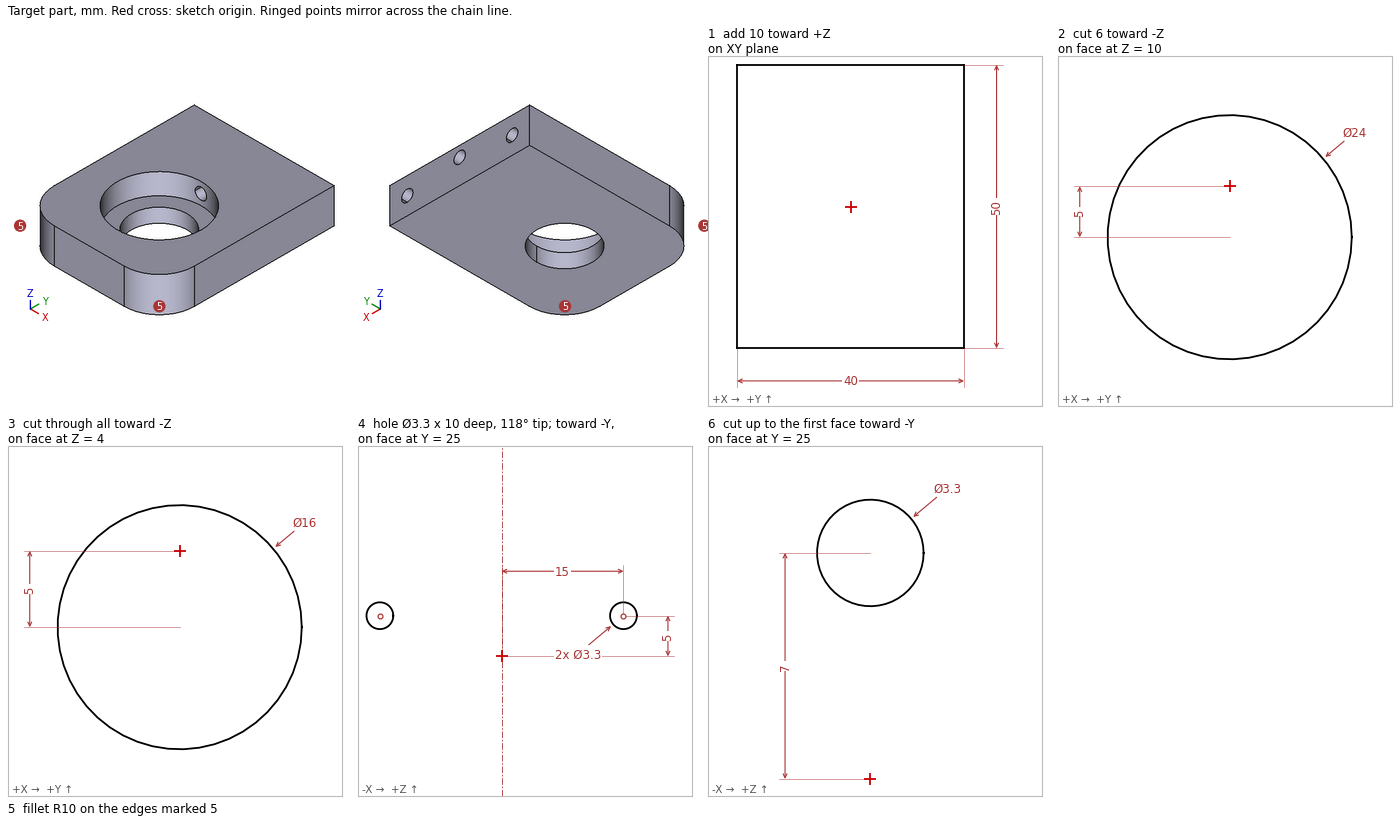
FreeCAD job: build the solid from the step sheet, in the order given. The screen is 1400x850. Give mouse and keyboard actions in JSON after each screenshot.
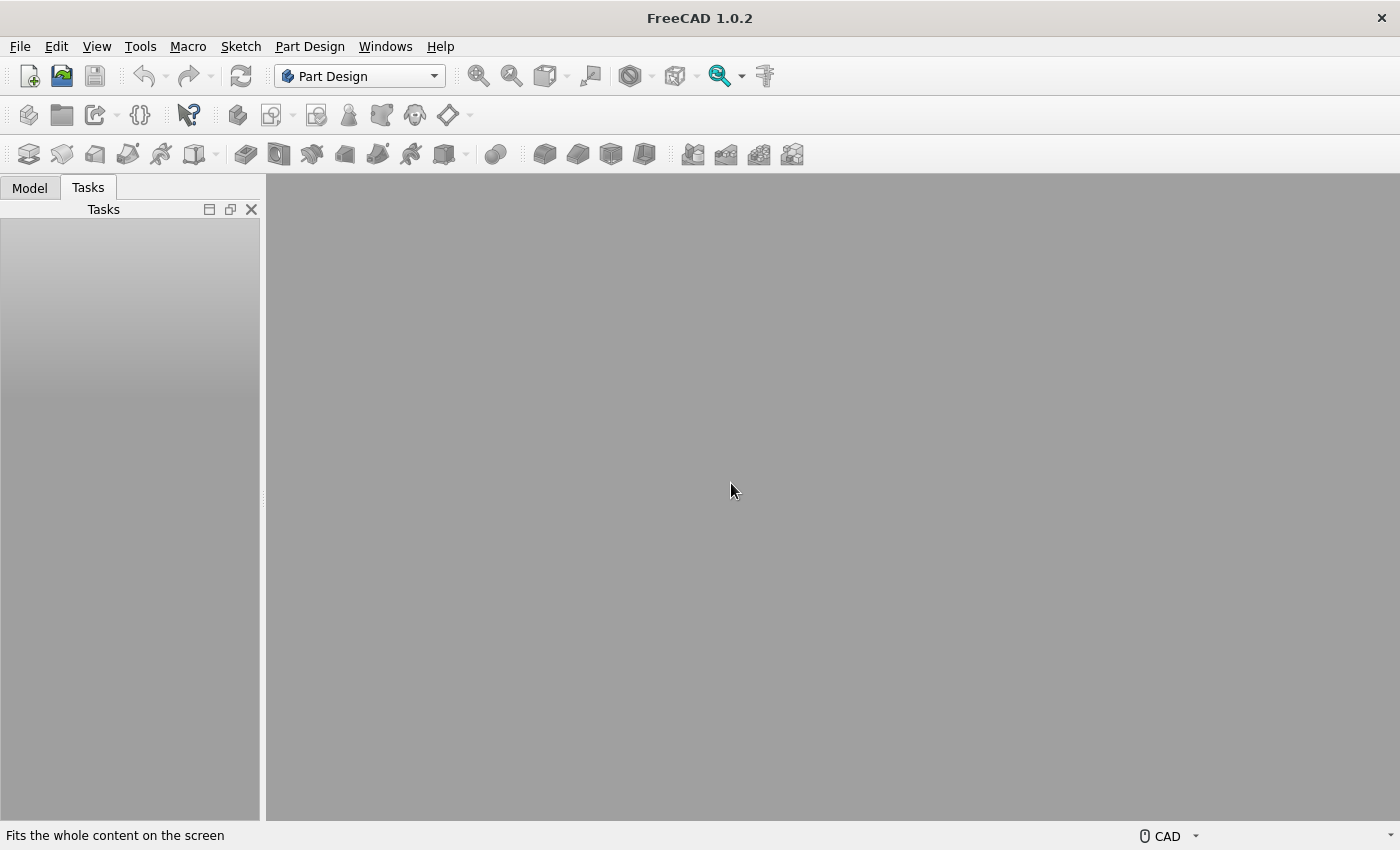
{"action": "left_click", "coordinate": [29, 76]}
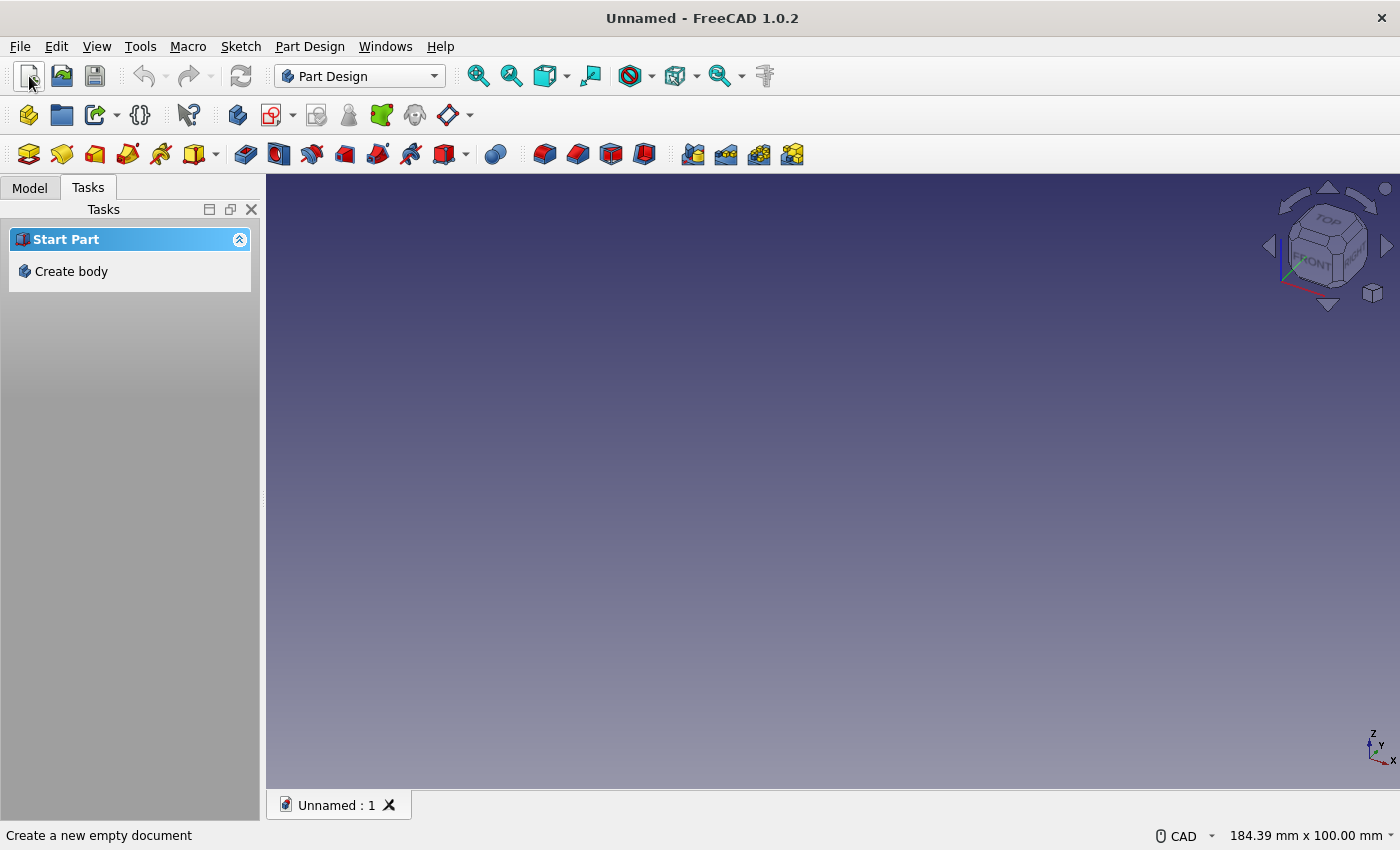
{"action": "left_click", "coordinate": [270, 116]}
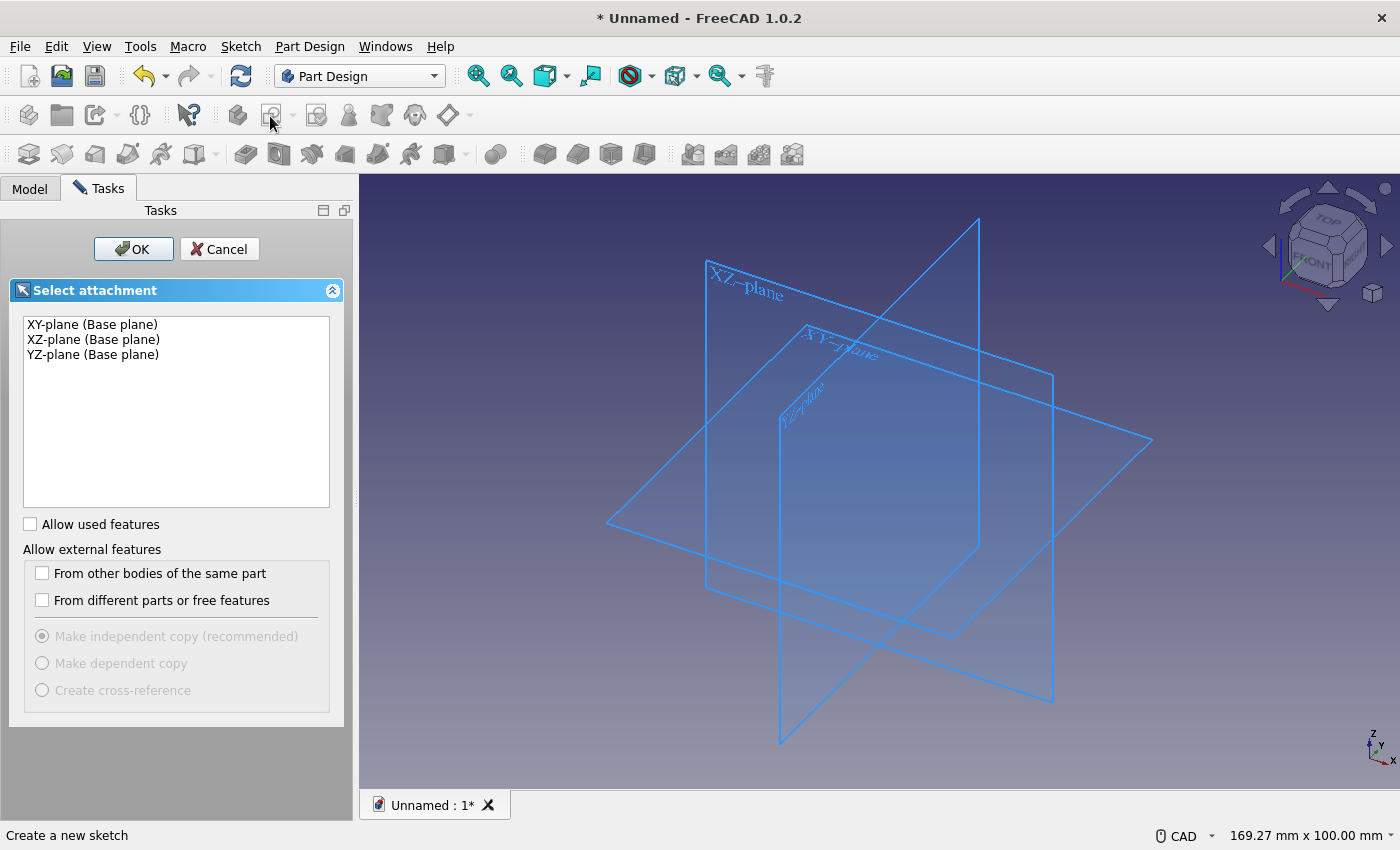
{"action": "left_click", "coordinate": [84, 324]}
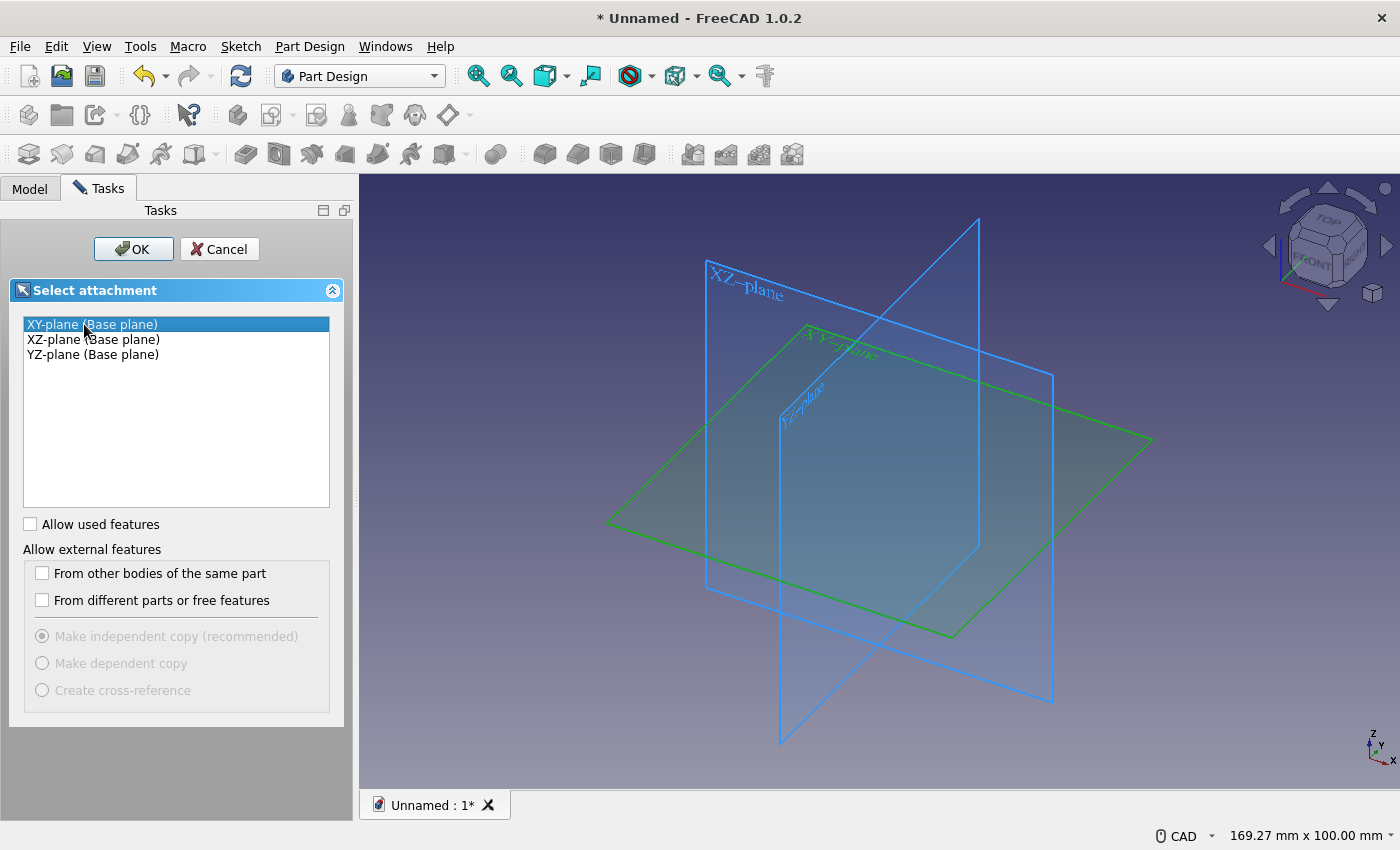
{"action": "left_click", "coordinate": [134, 249]}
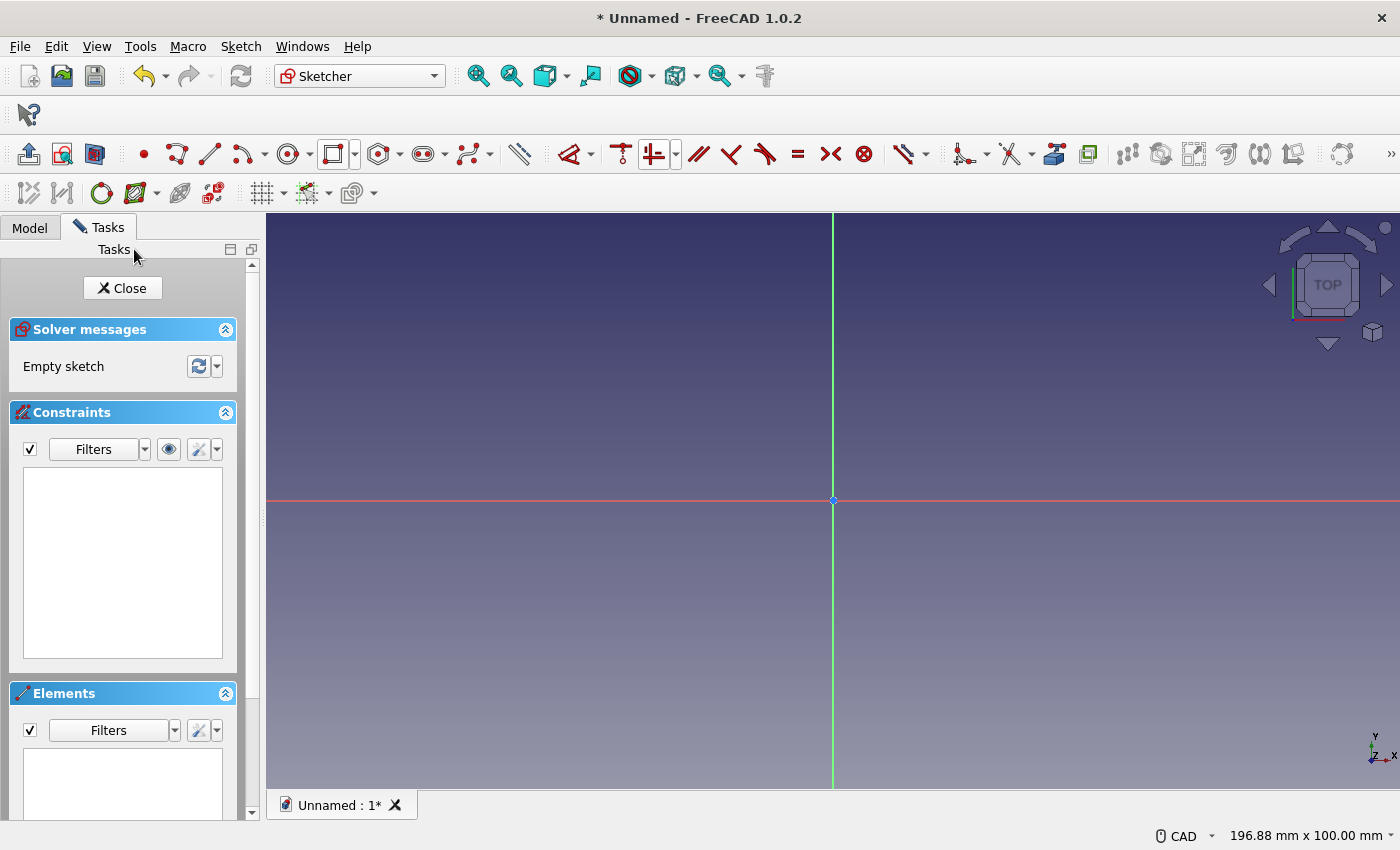
{"action": "key", "text": "g v"}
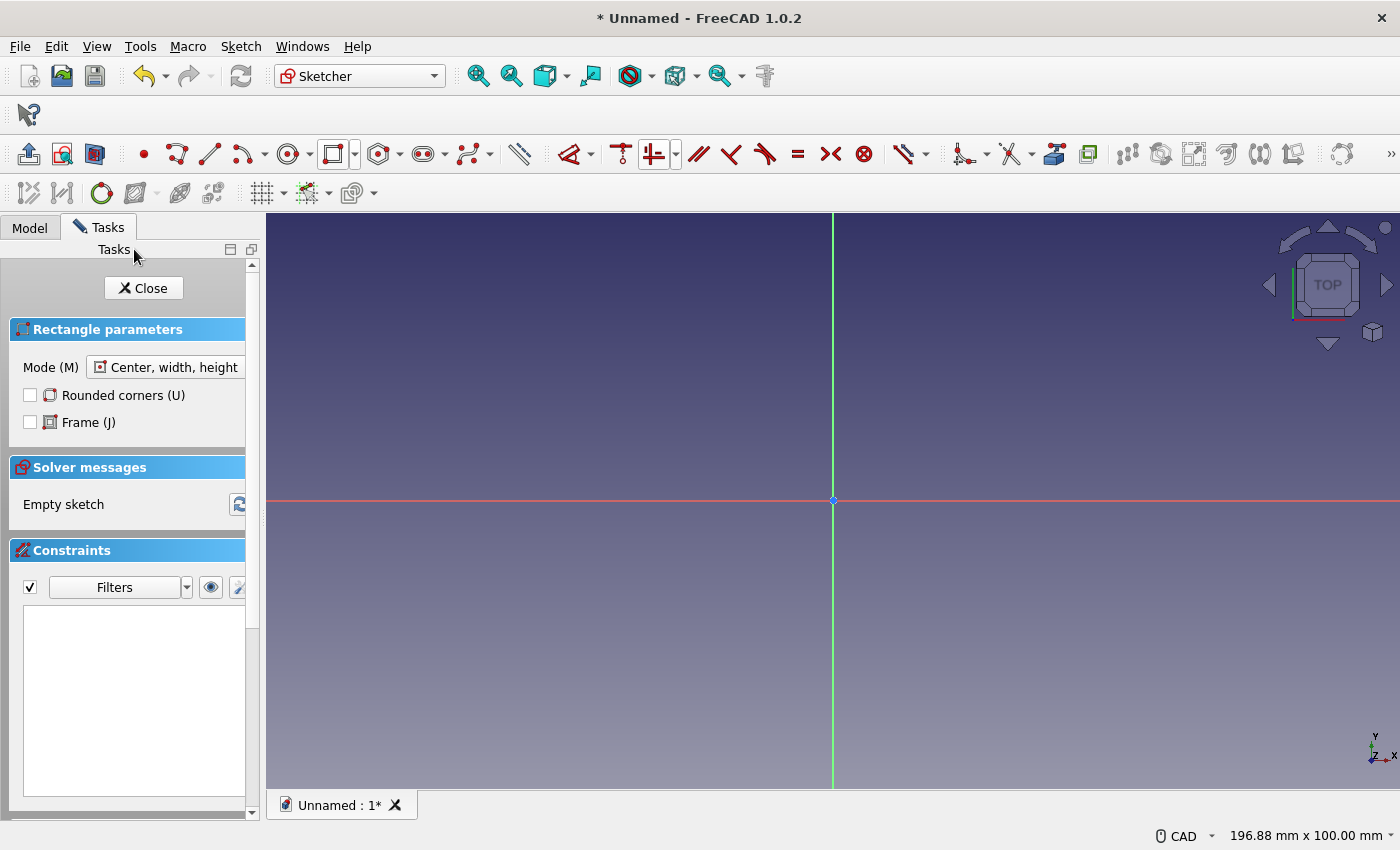
{"action": "left_click", "coordinate": [833, 501]}
{"action": "mouse_move", "coordinate": [948, 357]}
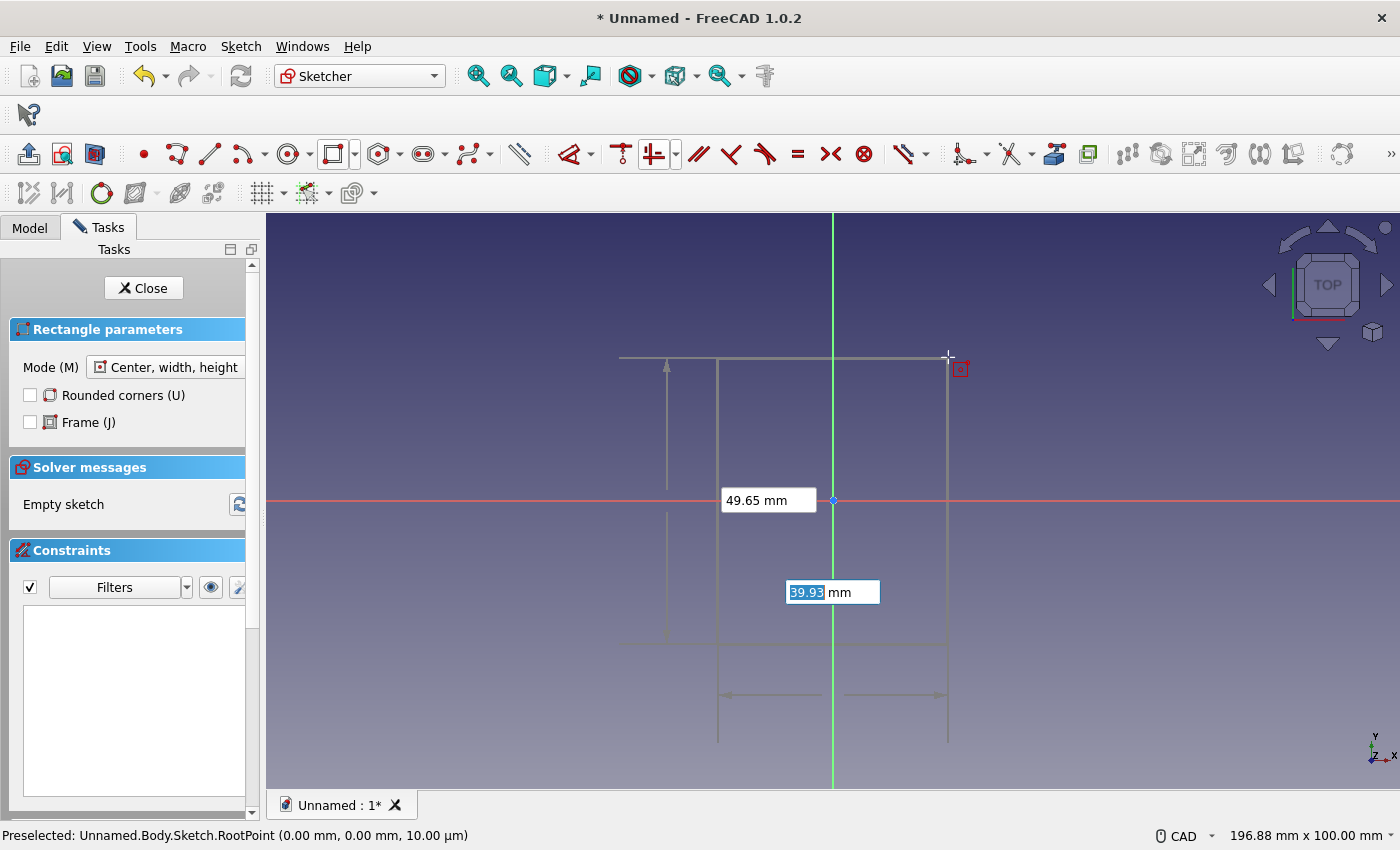
{"action": "type", "text": "40"}
{"action": "key", "text": "Tab"}
{"action": "type", "text": "50"}
{"action": "key", "text": "Return"}
{"action": "key", "text": "Escape"}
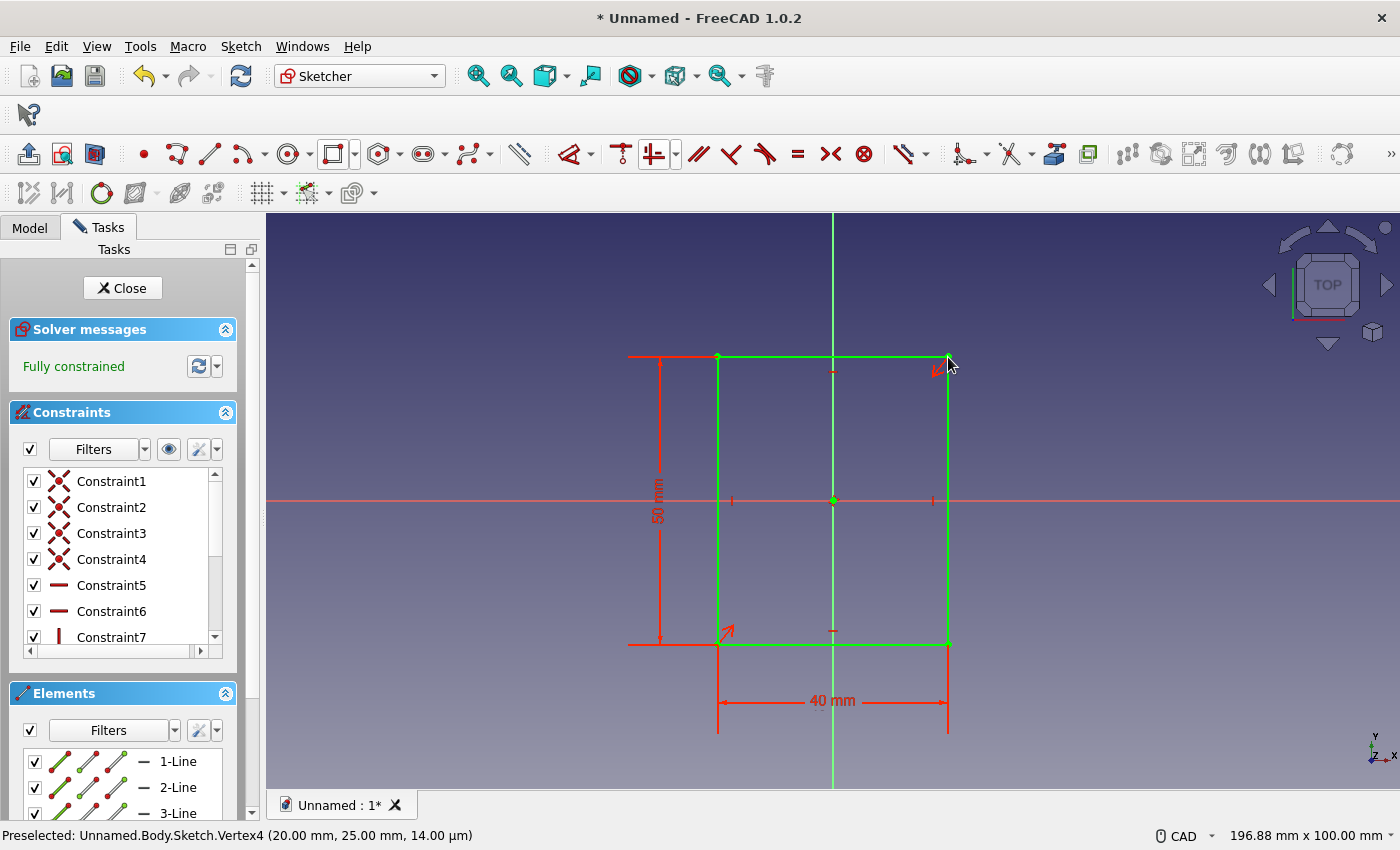
{"action": "left_click", "coordinate": [123, 288]}